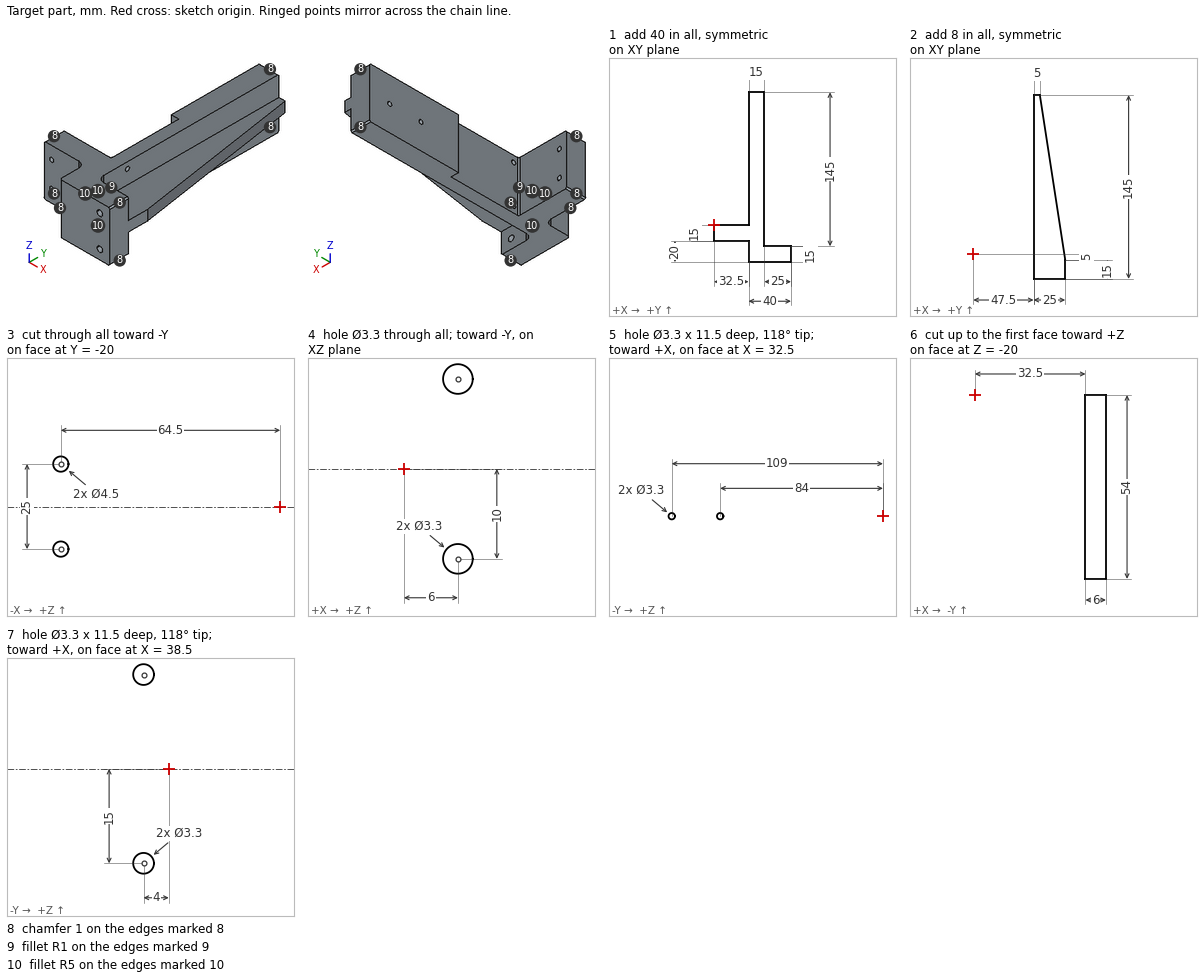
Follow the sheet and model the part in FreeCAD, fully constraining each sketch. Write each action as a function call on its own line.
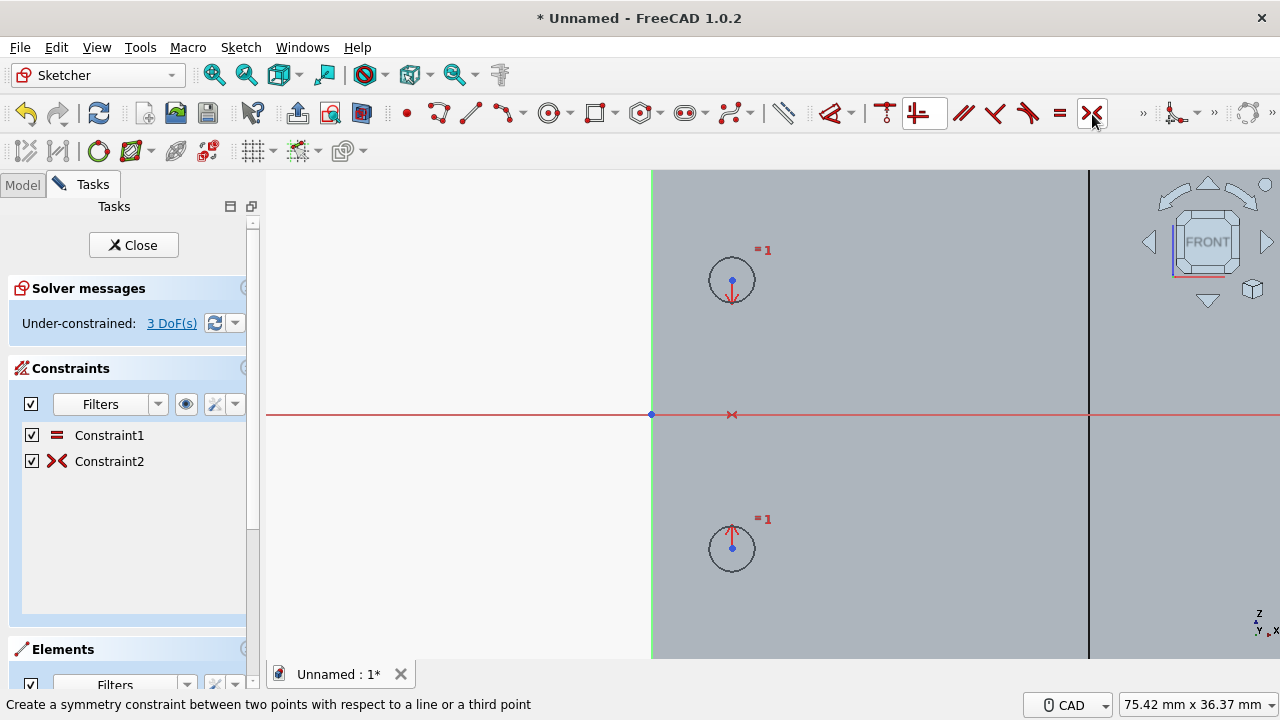
click(830, 114)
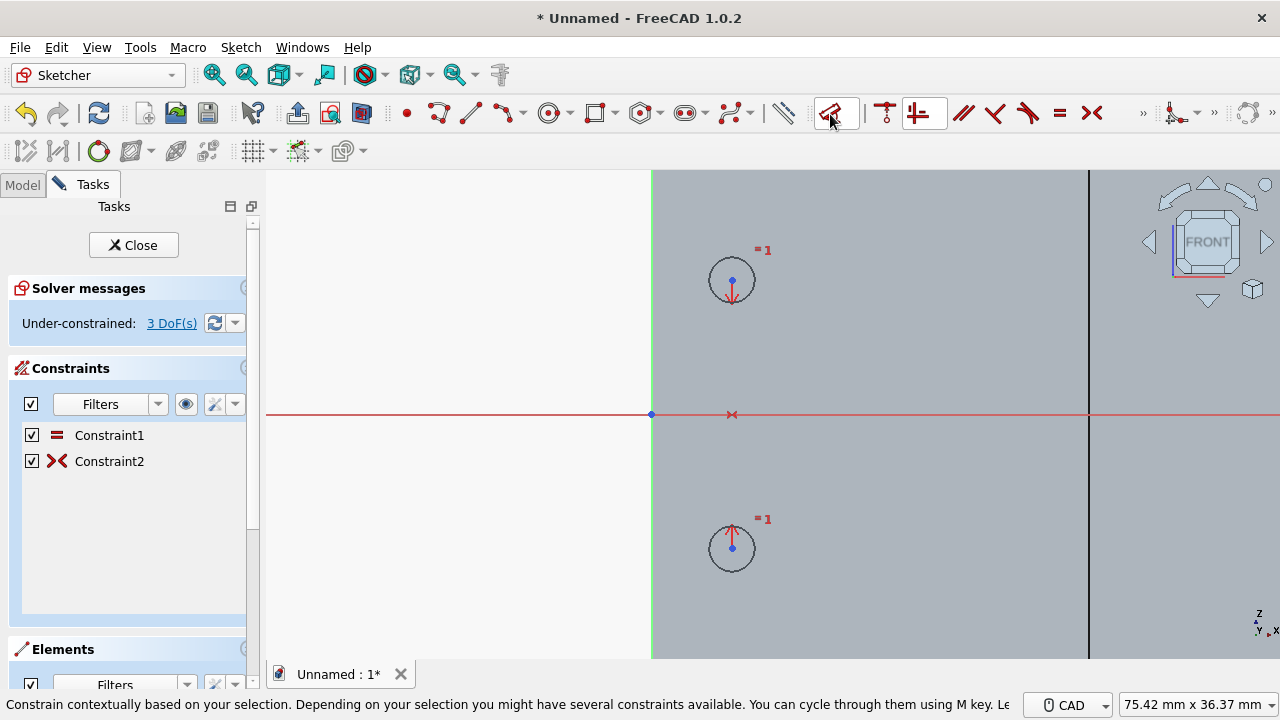
click(748, 533)
click(771, 510)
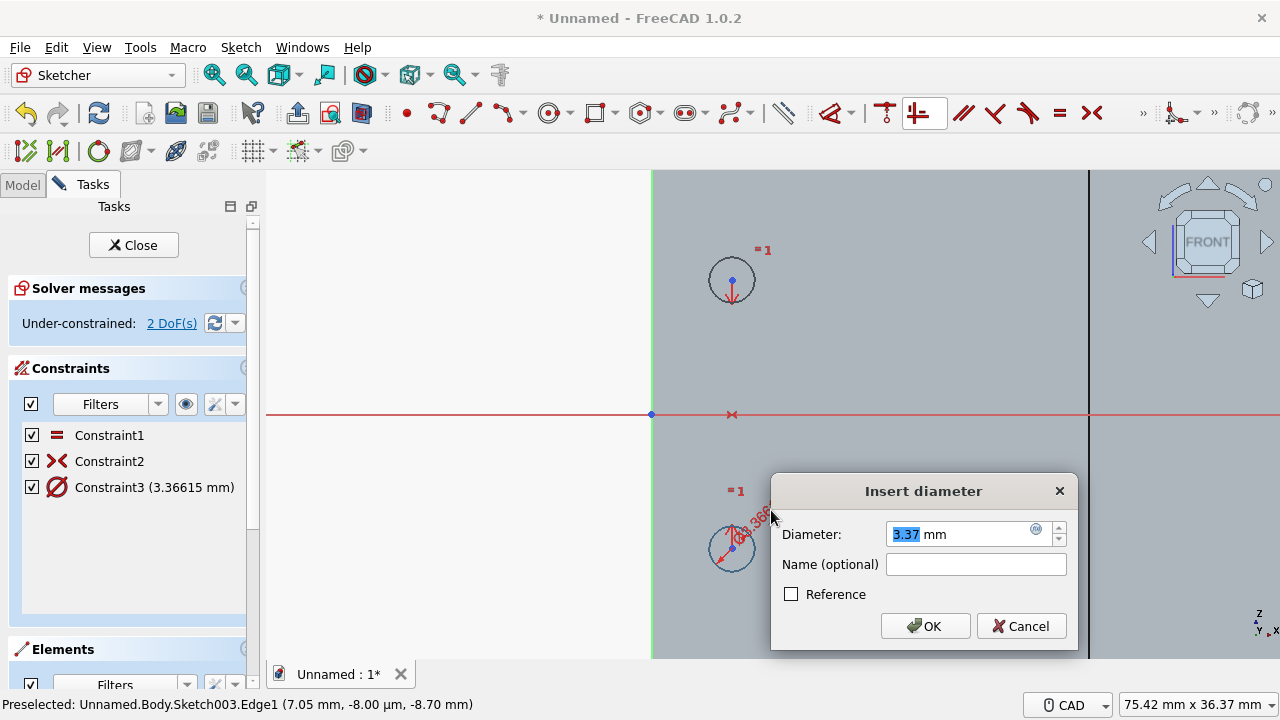
text(3.3)
key(Return)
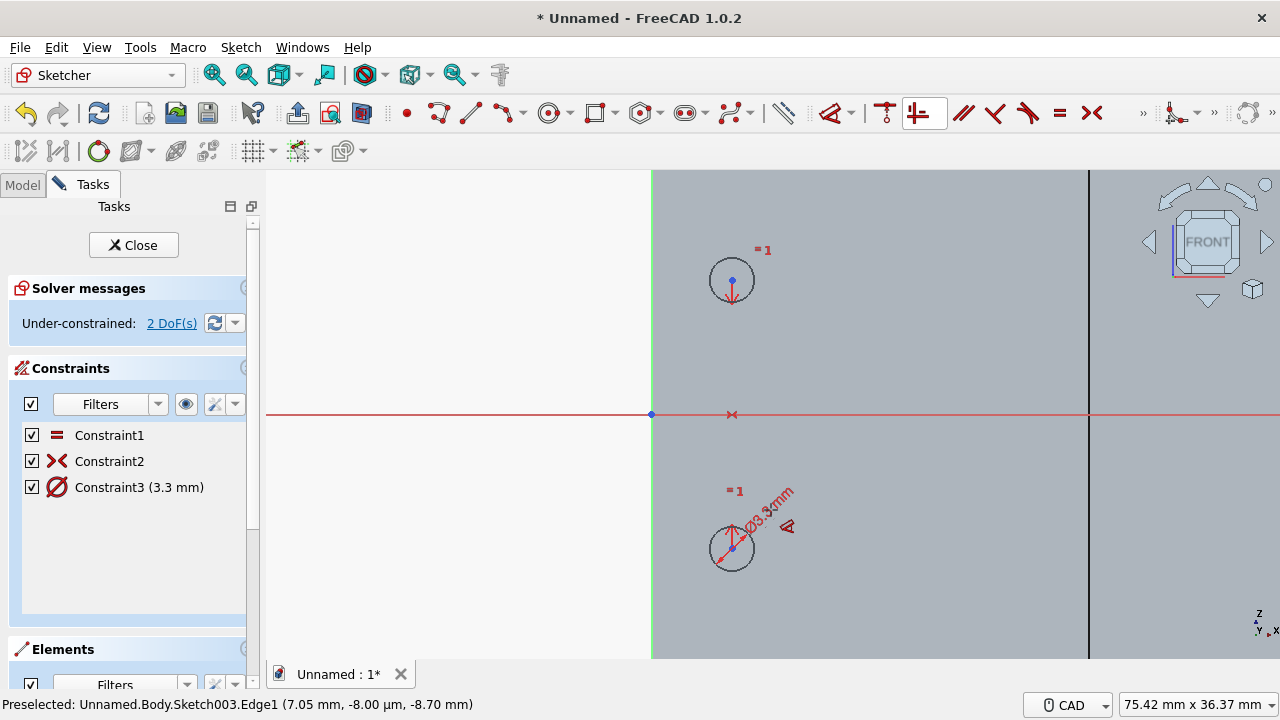
click(732, 549)
click(692, 583)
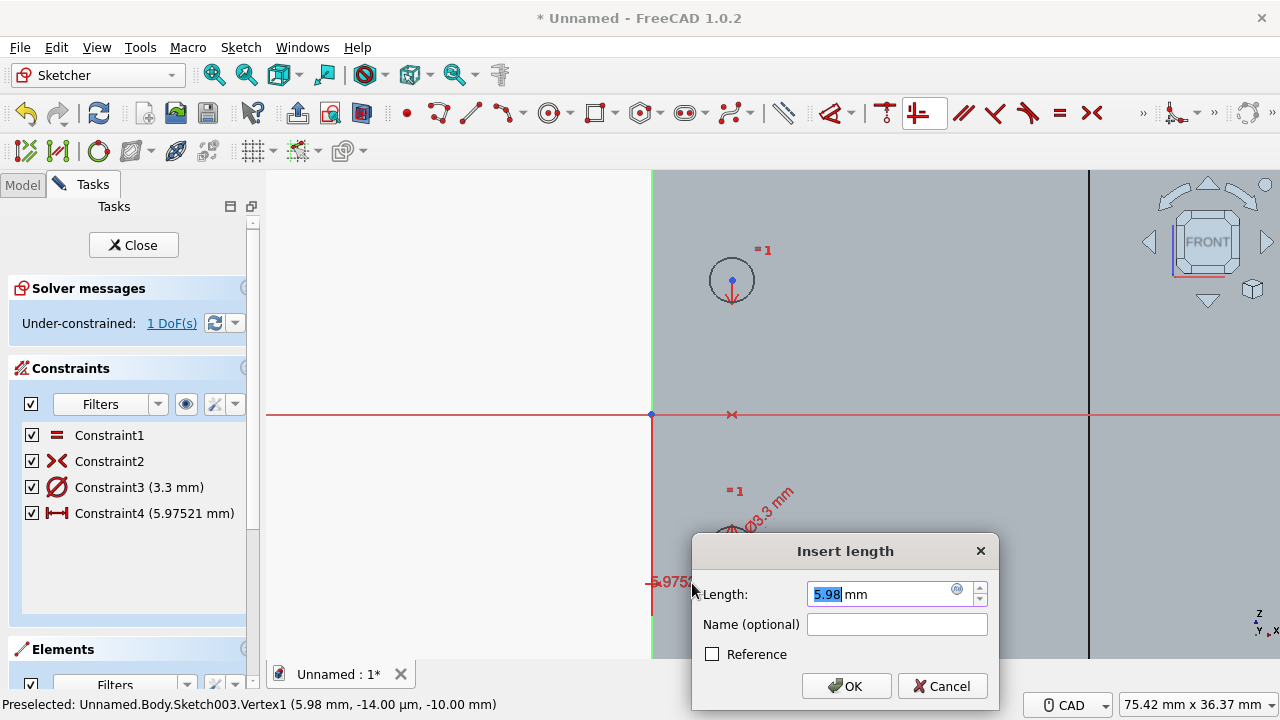
text(6)
key(Return)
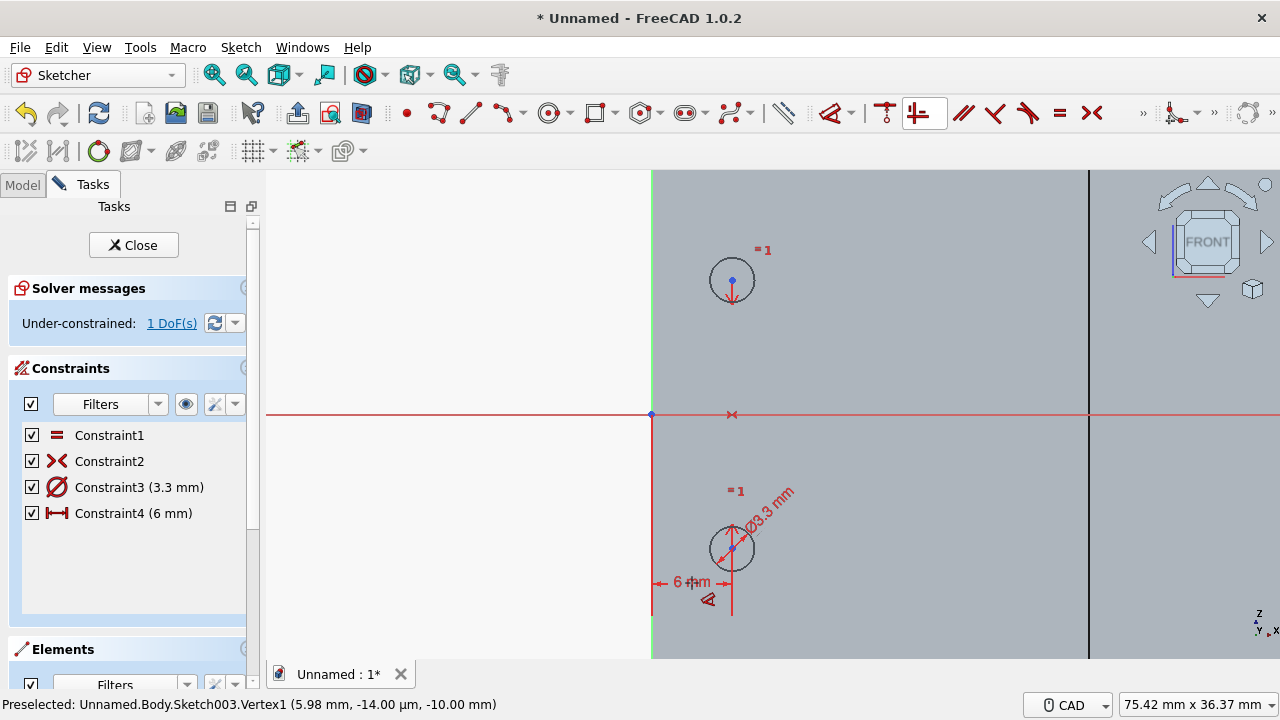
click(732, 549)
click(618, 482)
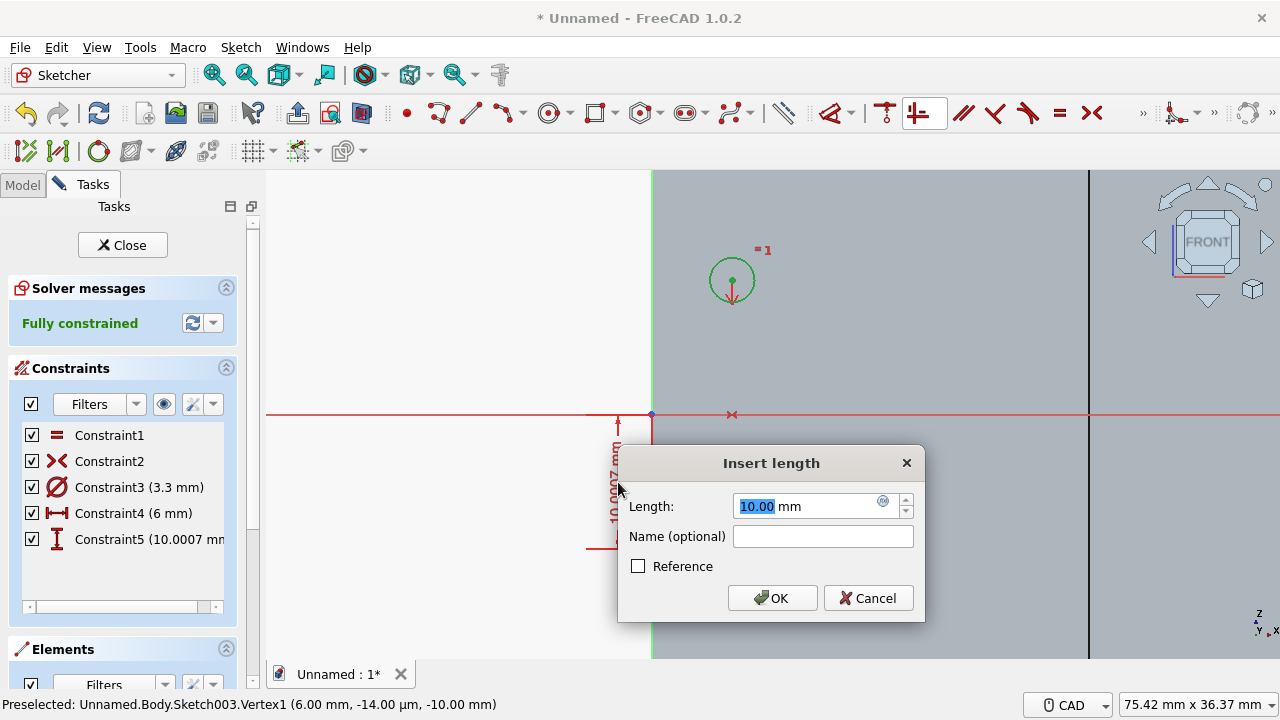
text(10)
key(Return)
key(Escape)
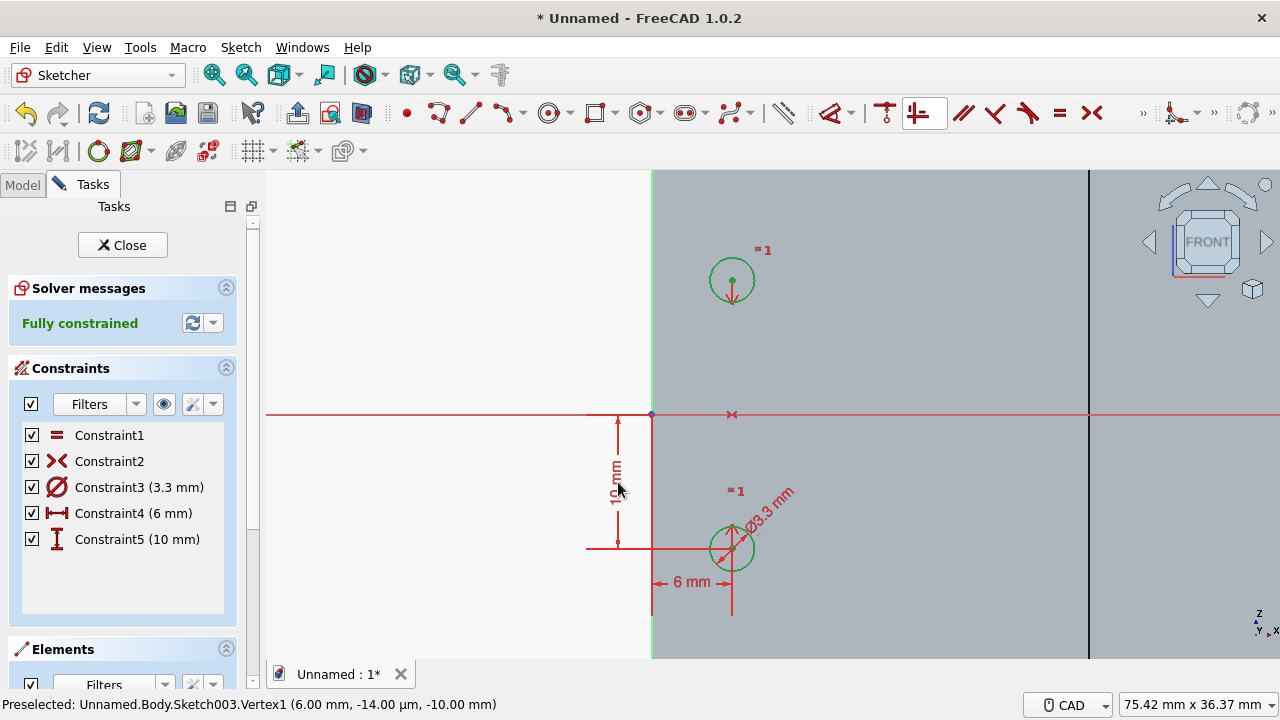
click(123, 245)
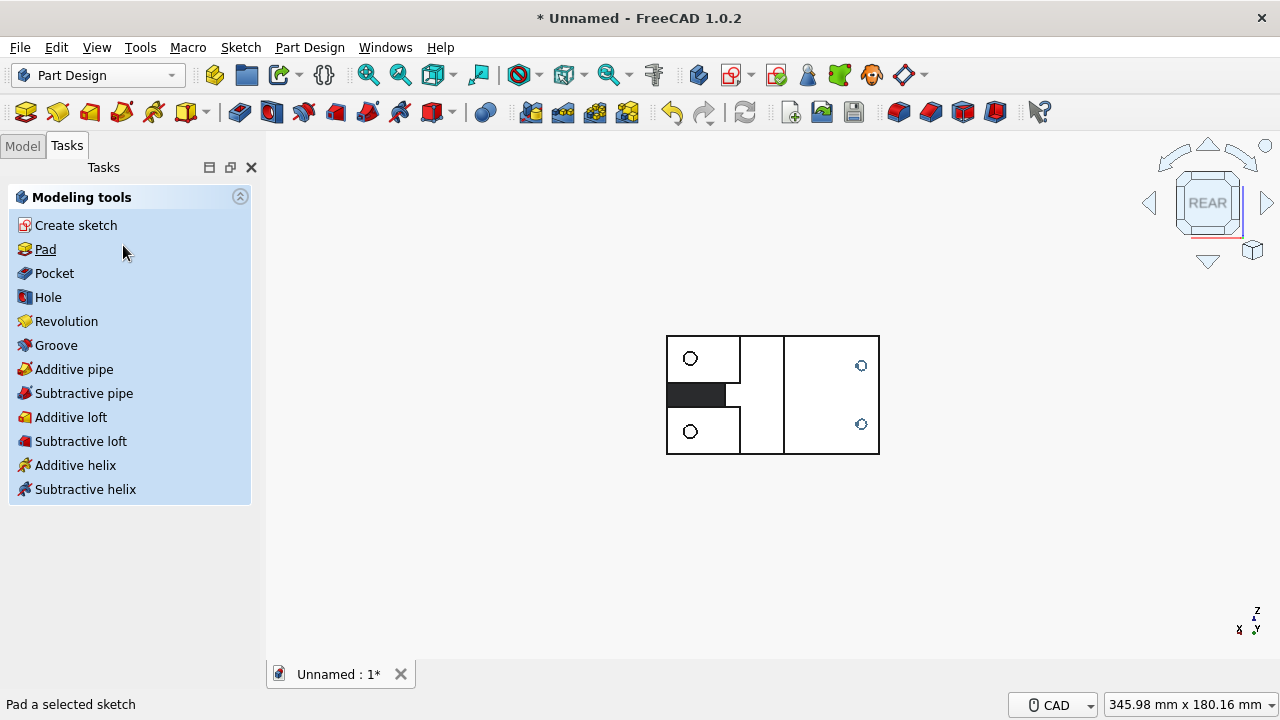
click(272, 112)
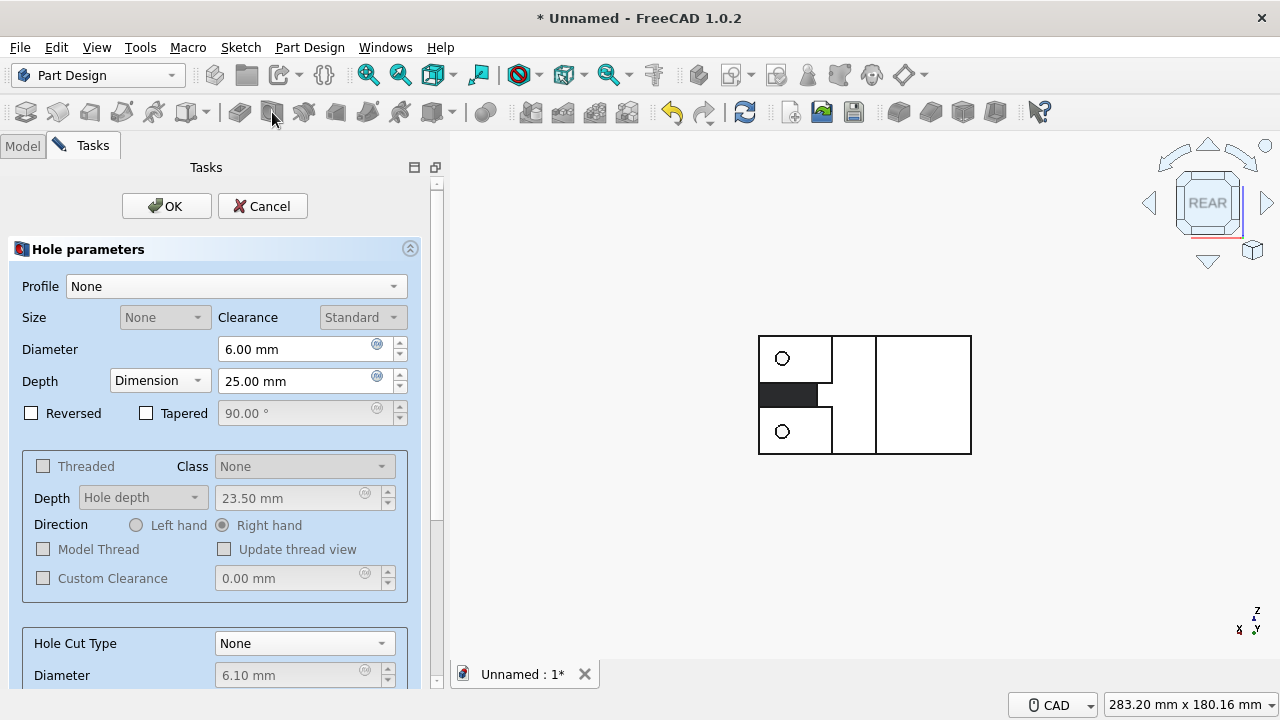
triple_click(305, 349)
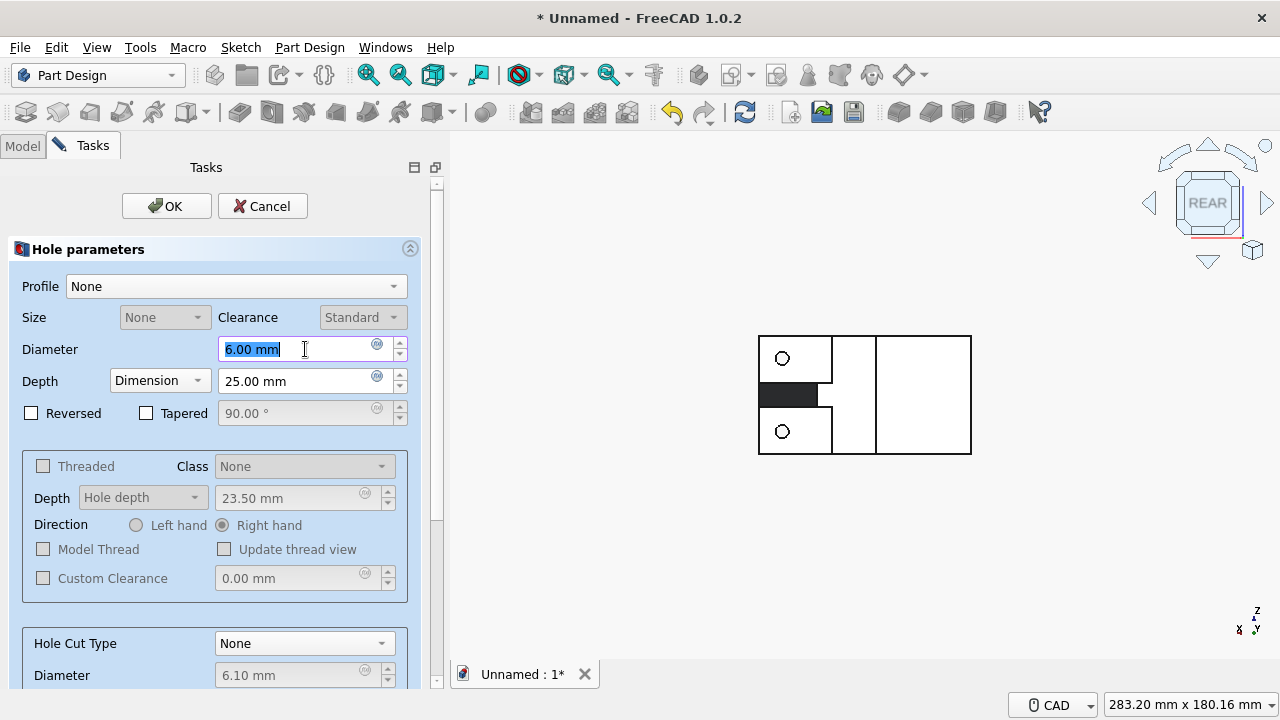
text(3.3)
key(Tab)